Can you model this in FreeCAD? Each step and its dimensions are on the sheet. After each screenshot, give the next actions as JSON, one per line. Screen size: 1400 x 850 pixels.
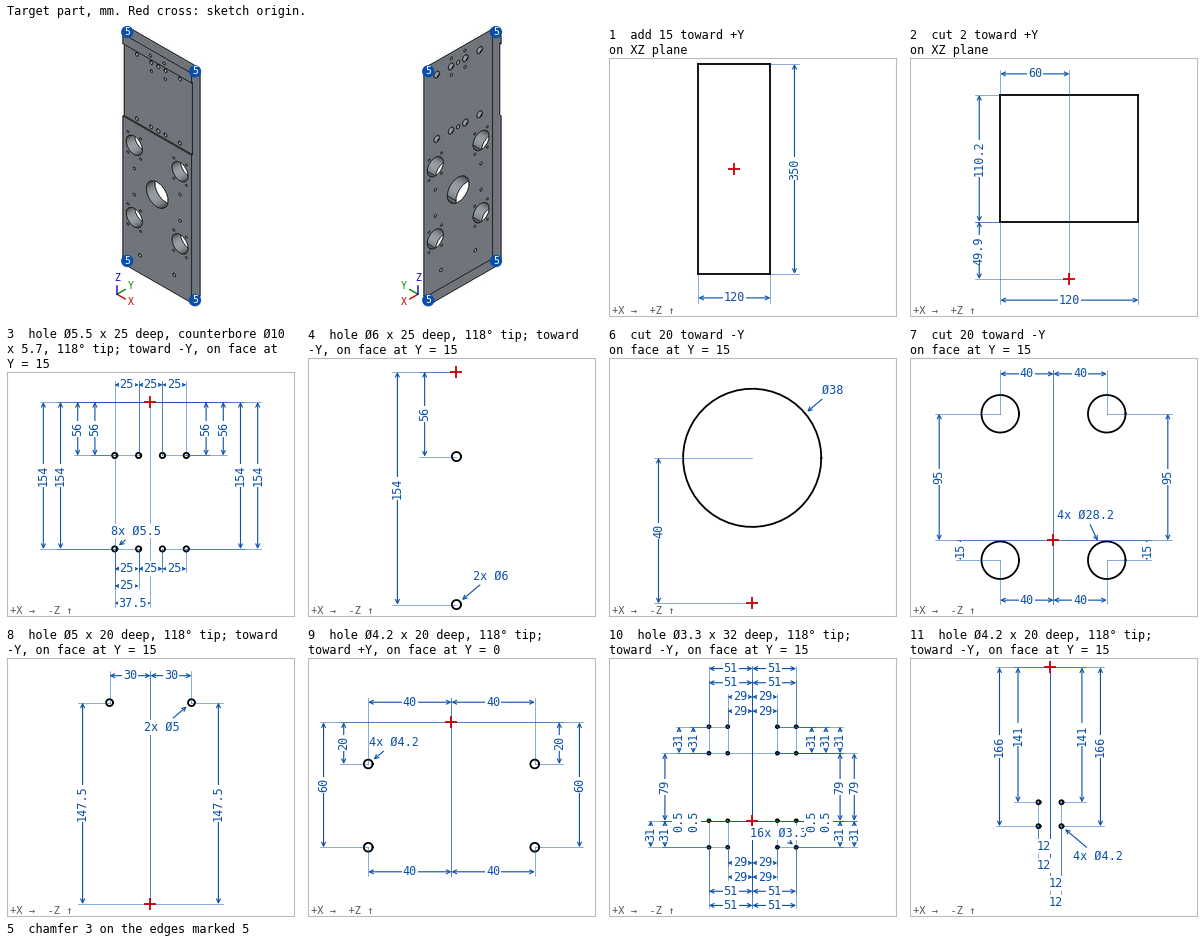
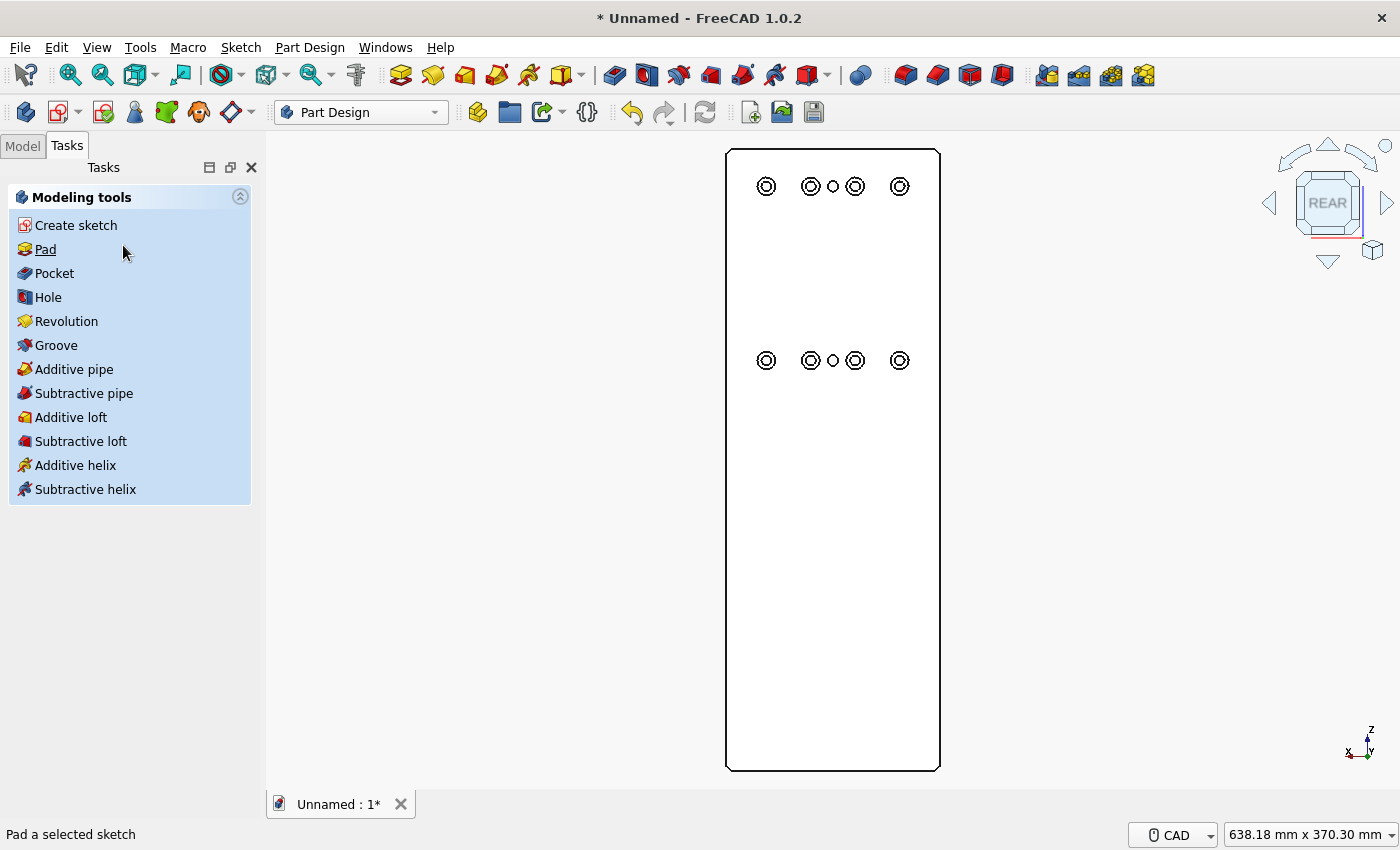
{"action": "left_click", "coordinate": [616, 76]}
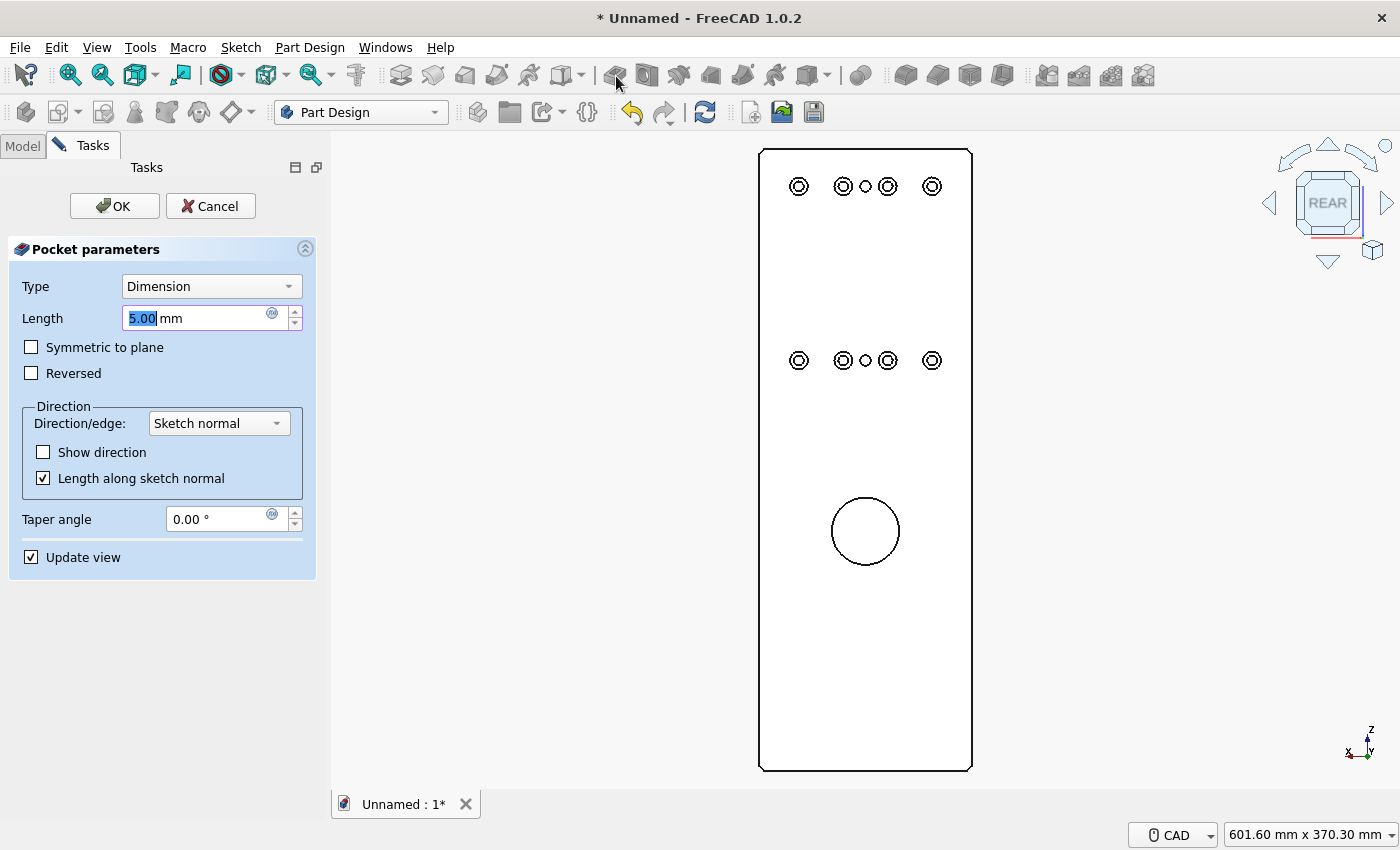
{"action": "type", "text": "20"}
{"action": "key", "text": "Tab"}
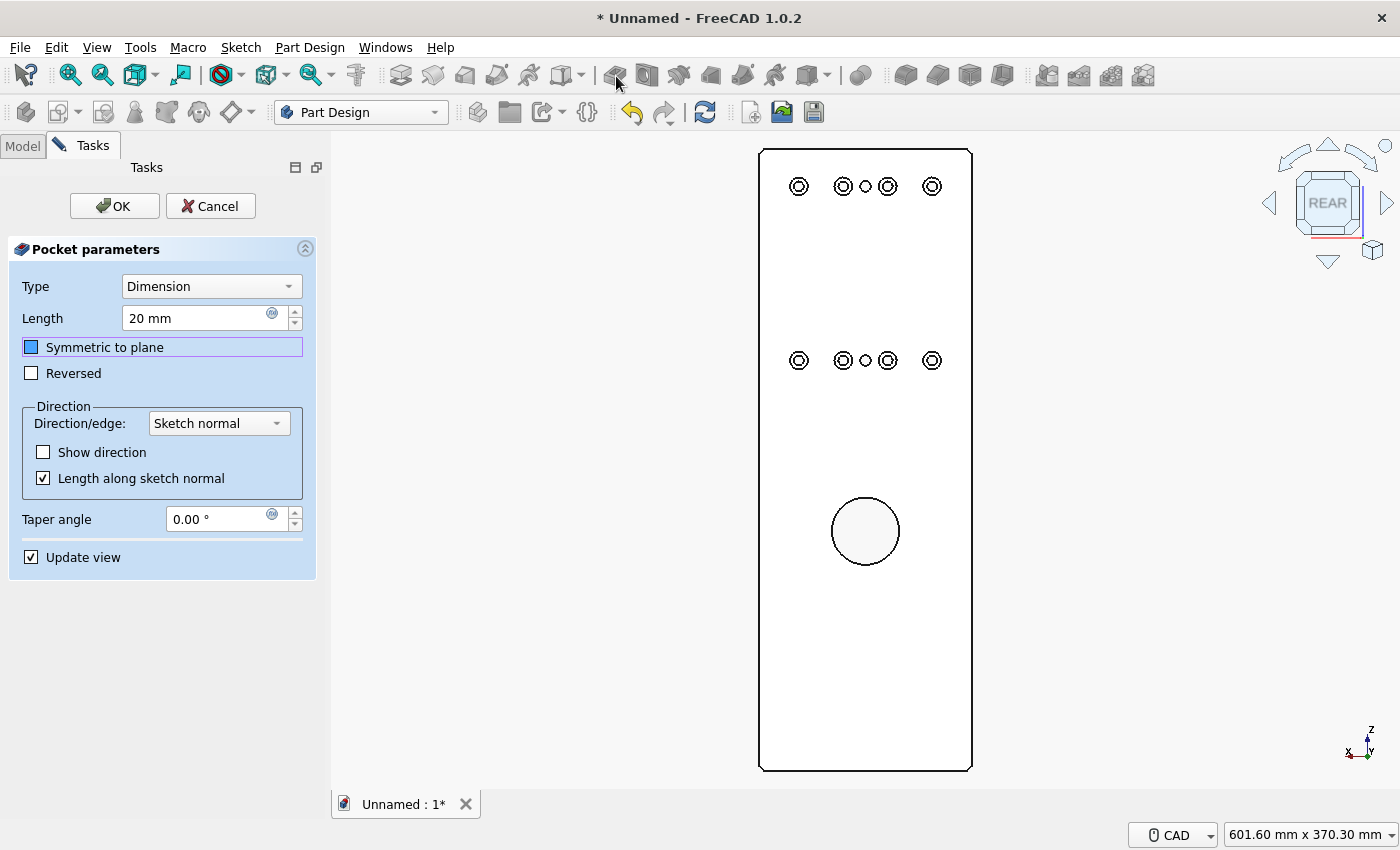
{"action": "left_click", "coordinate": [115, 206]}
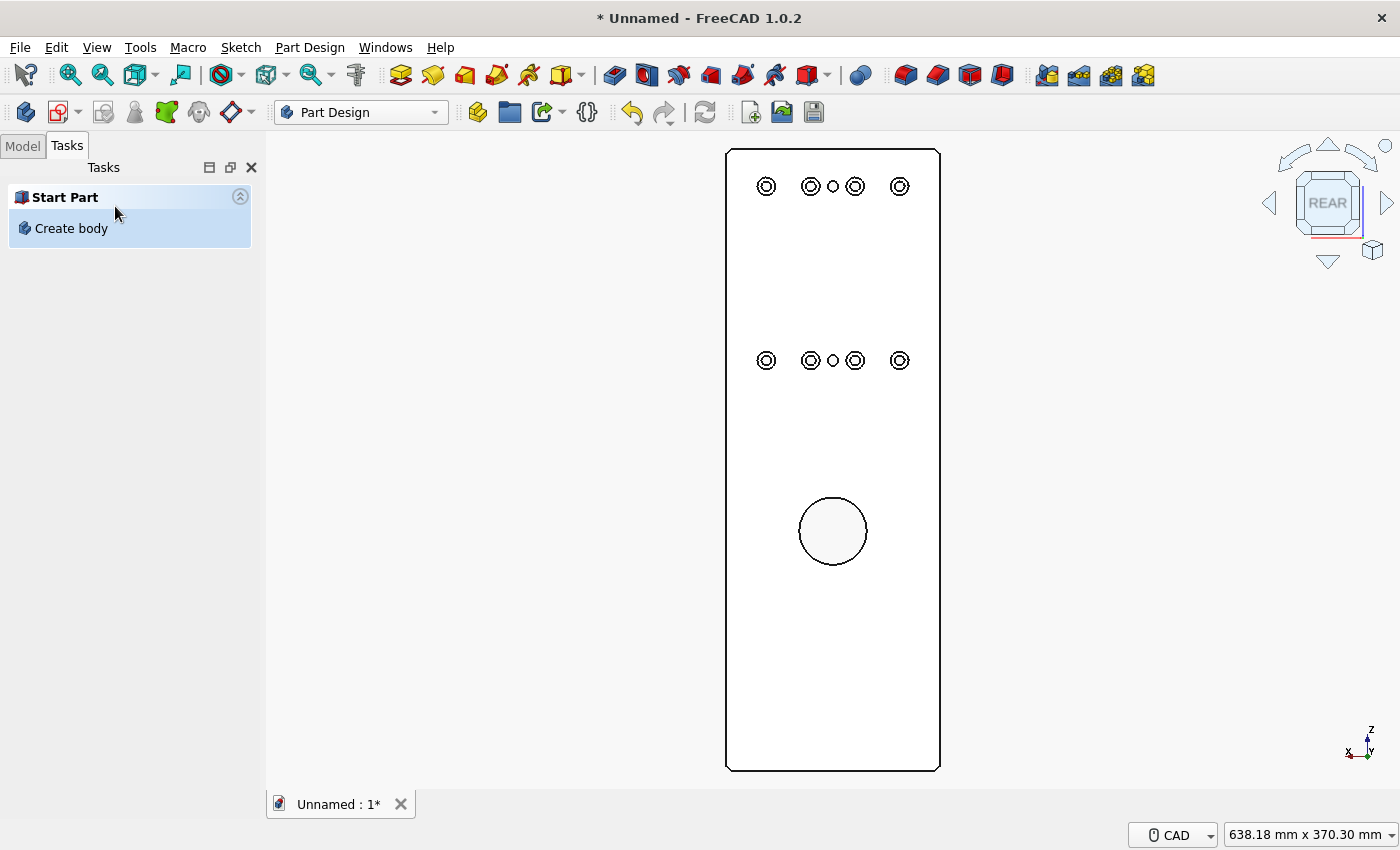
{"action": "left_click", "coordinate": [803, 637]}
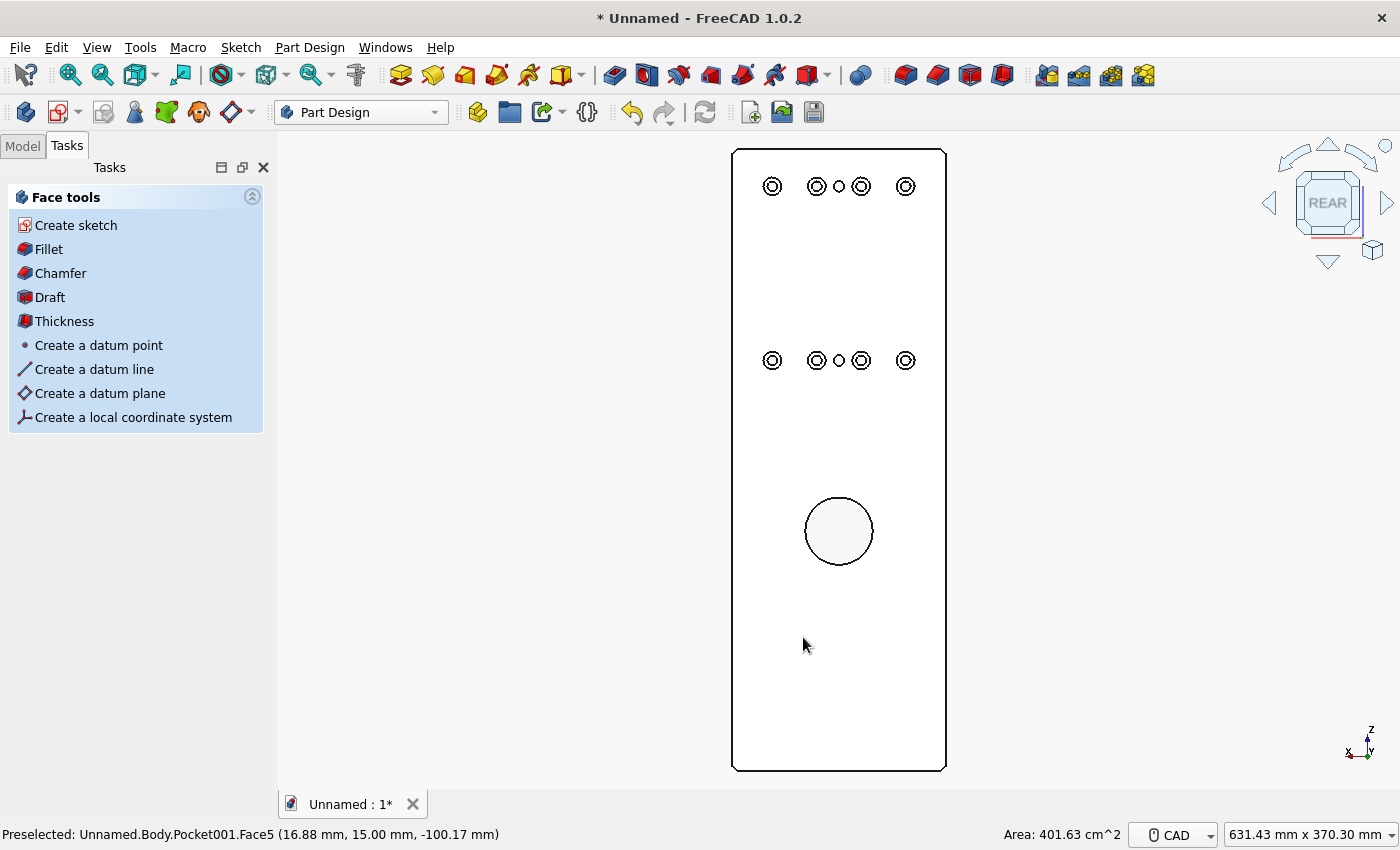
{"action": "left_click", "coordinate": [58, 112]}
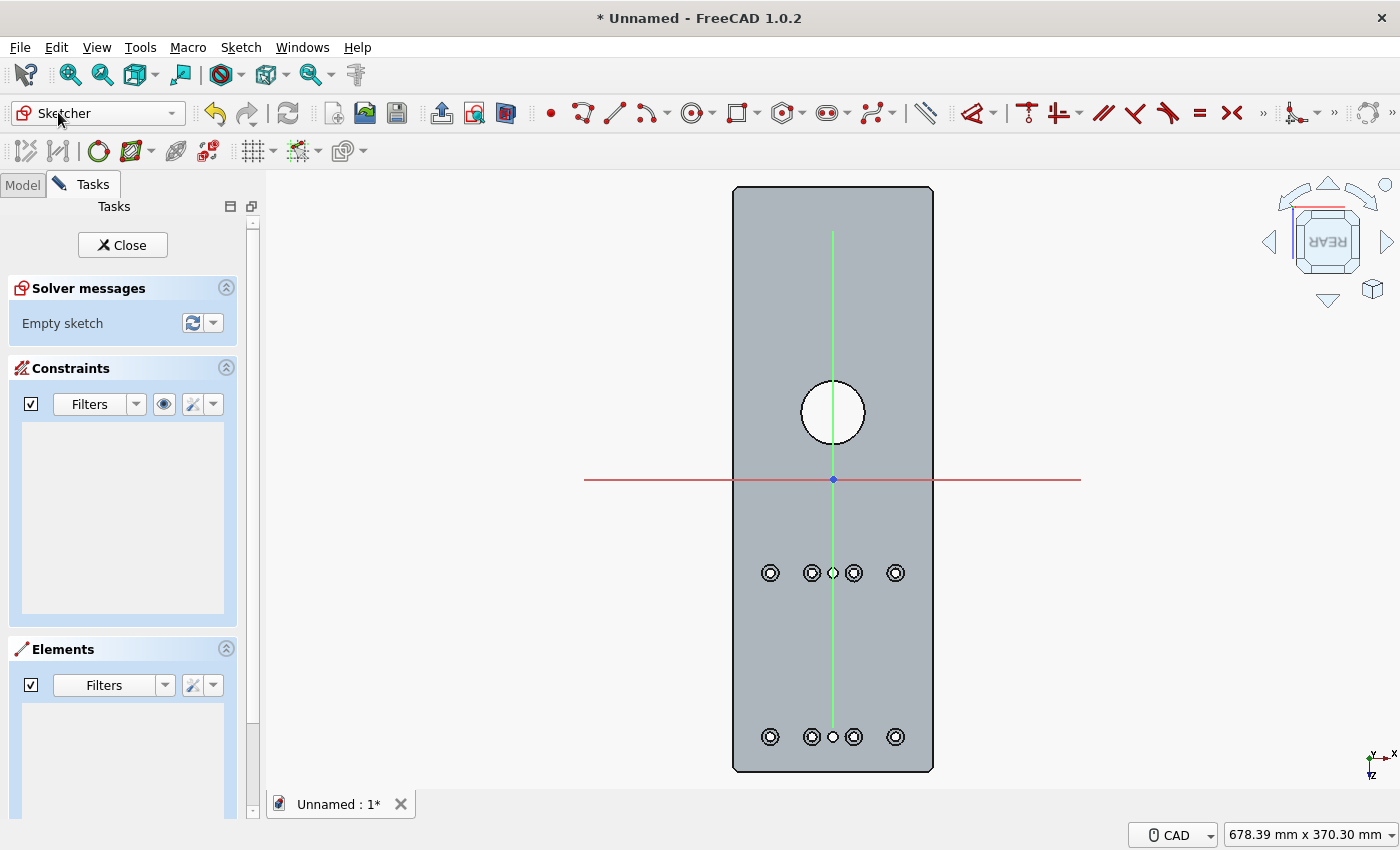
{"action": "scroll", "coordinate": [916, 331], "scroll_direction": "up", "scroll_amount": 3}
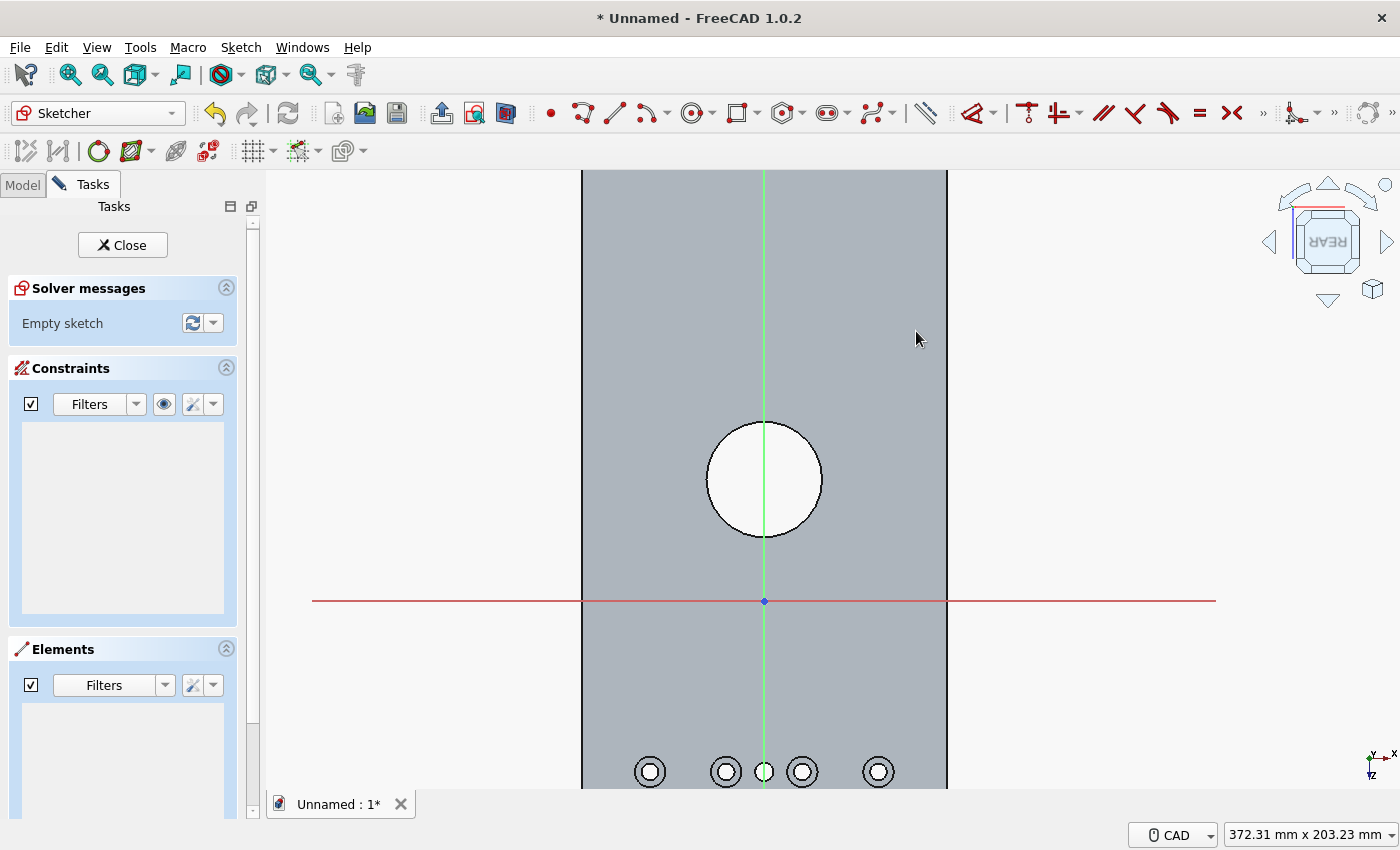
{"action": "key", "text": "g c"}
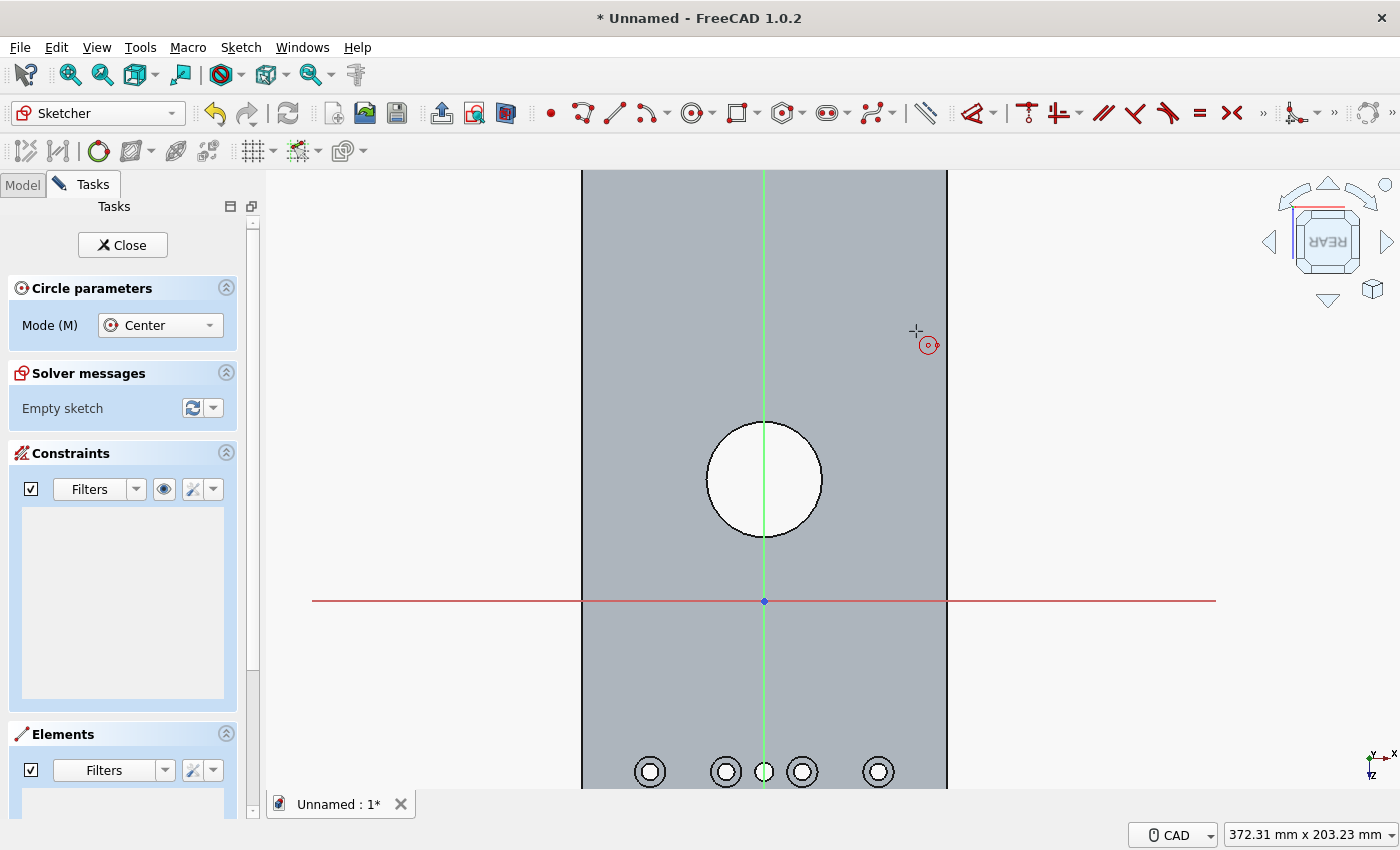
{"action": "left_click", "coordinate": [886, 647]}
{"action": "left_click", "coordinate": [916, 617]}